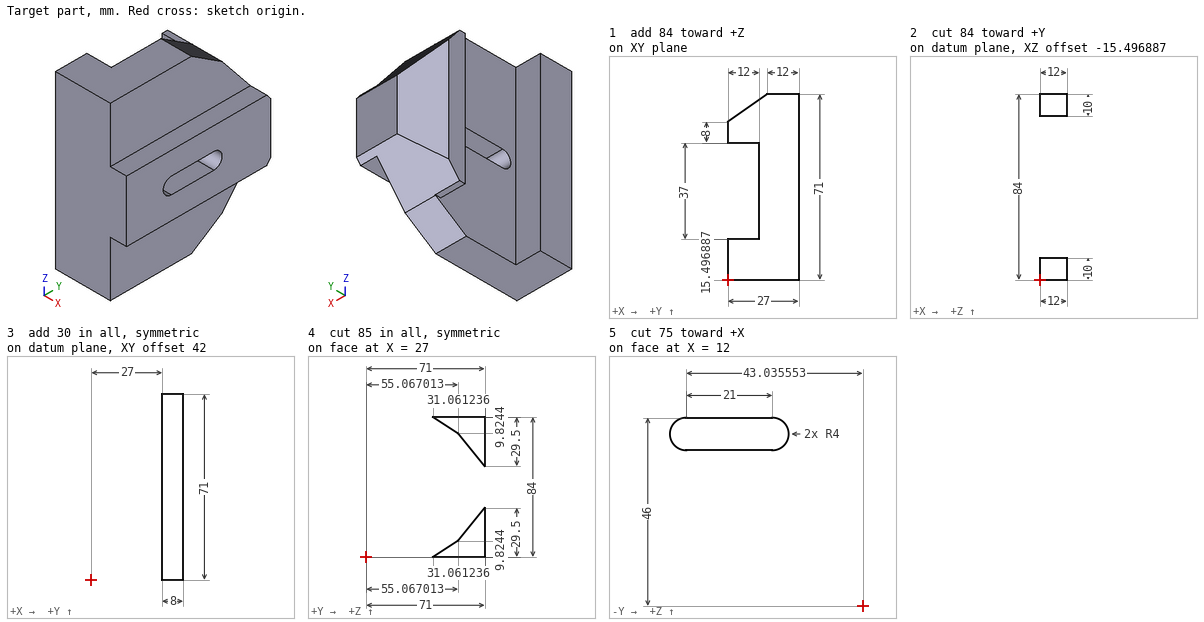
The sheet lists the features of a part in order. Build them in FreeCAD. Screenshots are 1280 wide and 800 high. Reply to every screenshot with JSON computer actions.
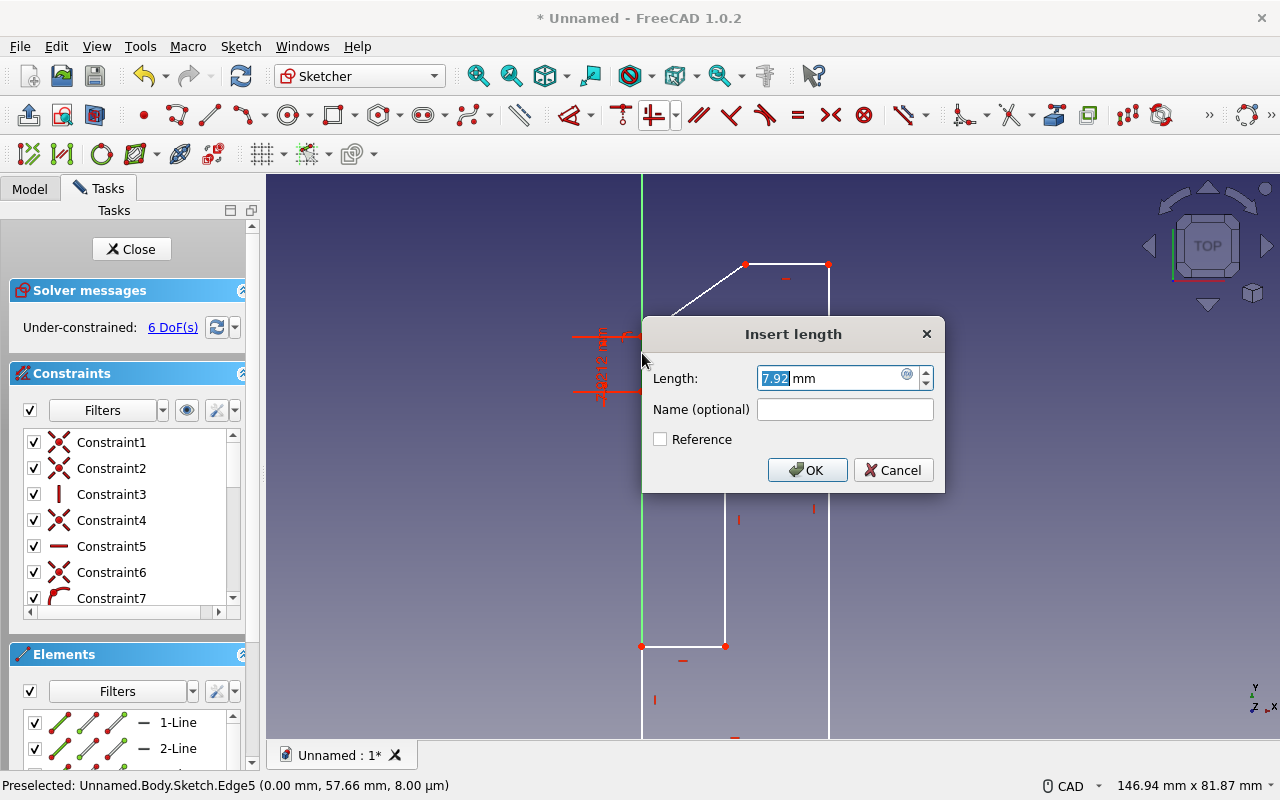
{"action": "type", "text": "8"}
{"action": "key", "text": "Return"}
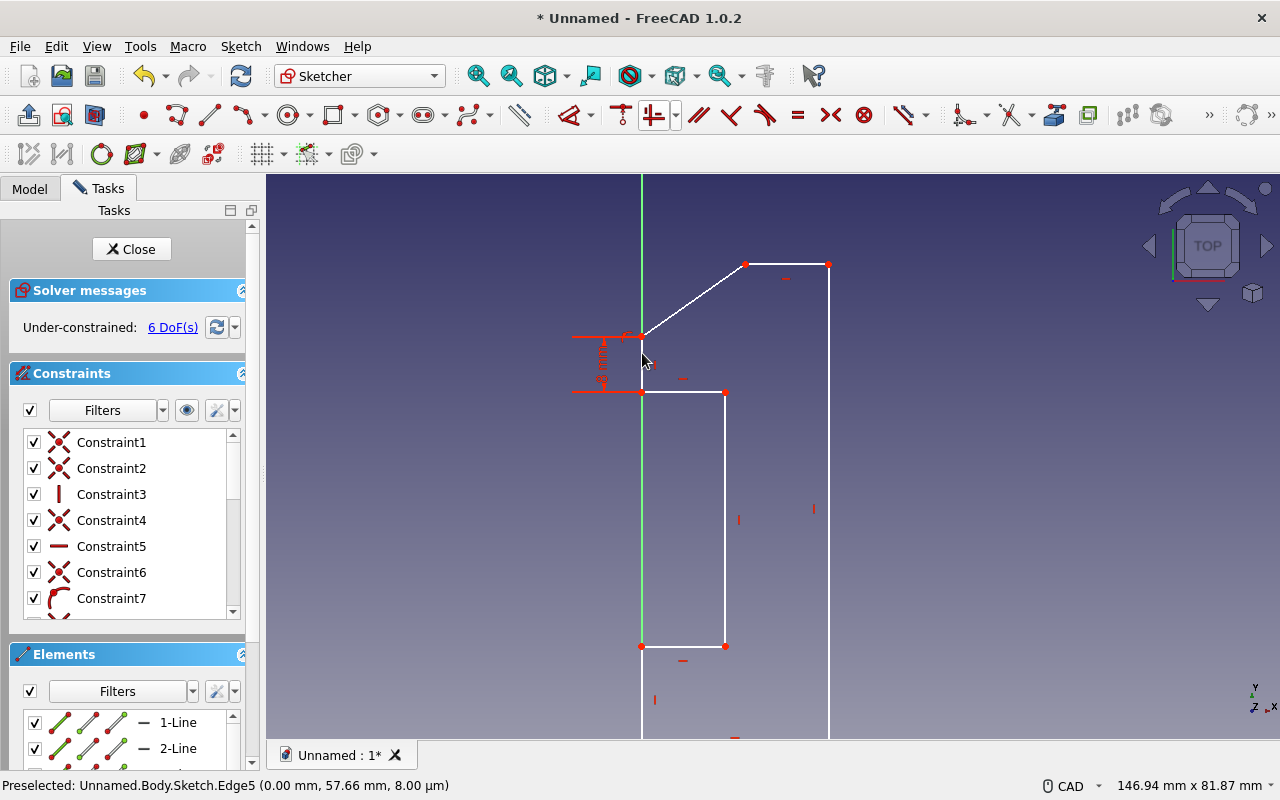
{"action": "scroll", "coordinate": [642, 354], "scroll_direction": "down", "scroll_amount": 2}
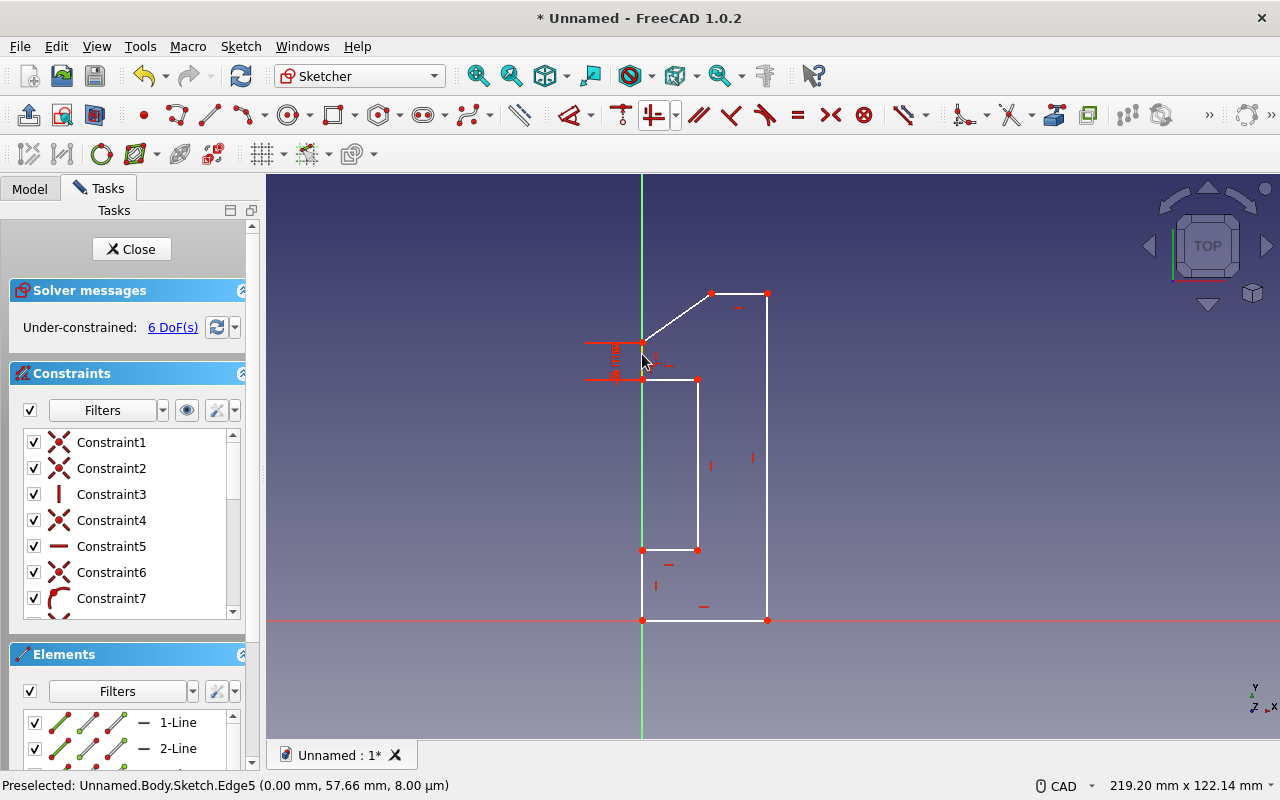
{"action": "left_click", "coordinate": [680, 621]}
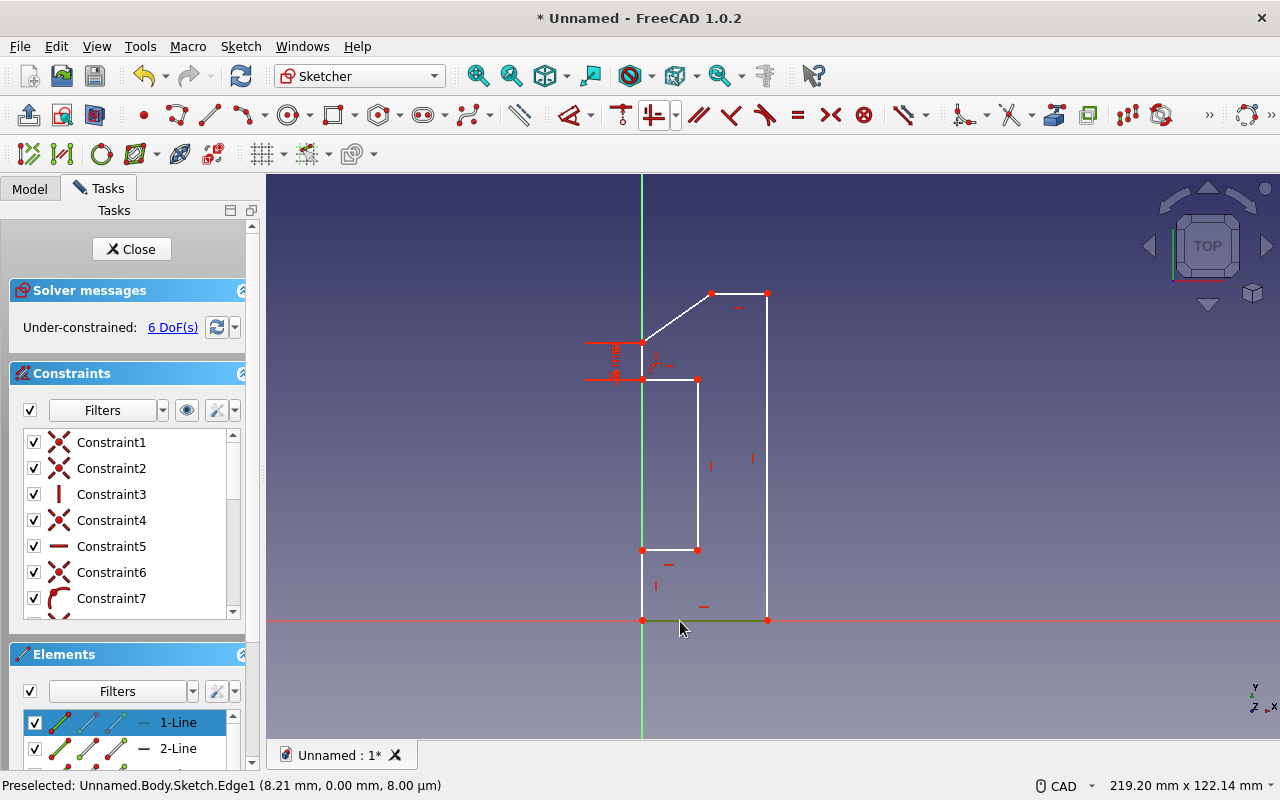
{"action": "key", "text": "l"}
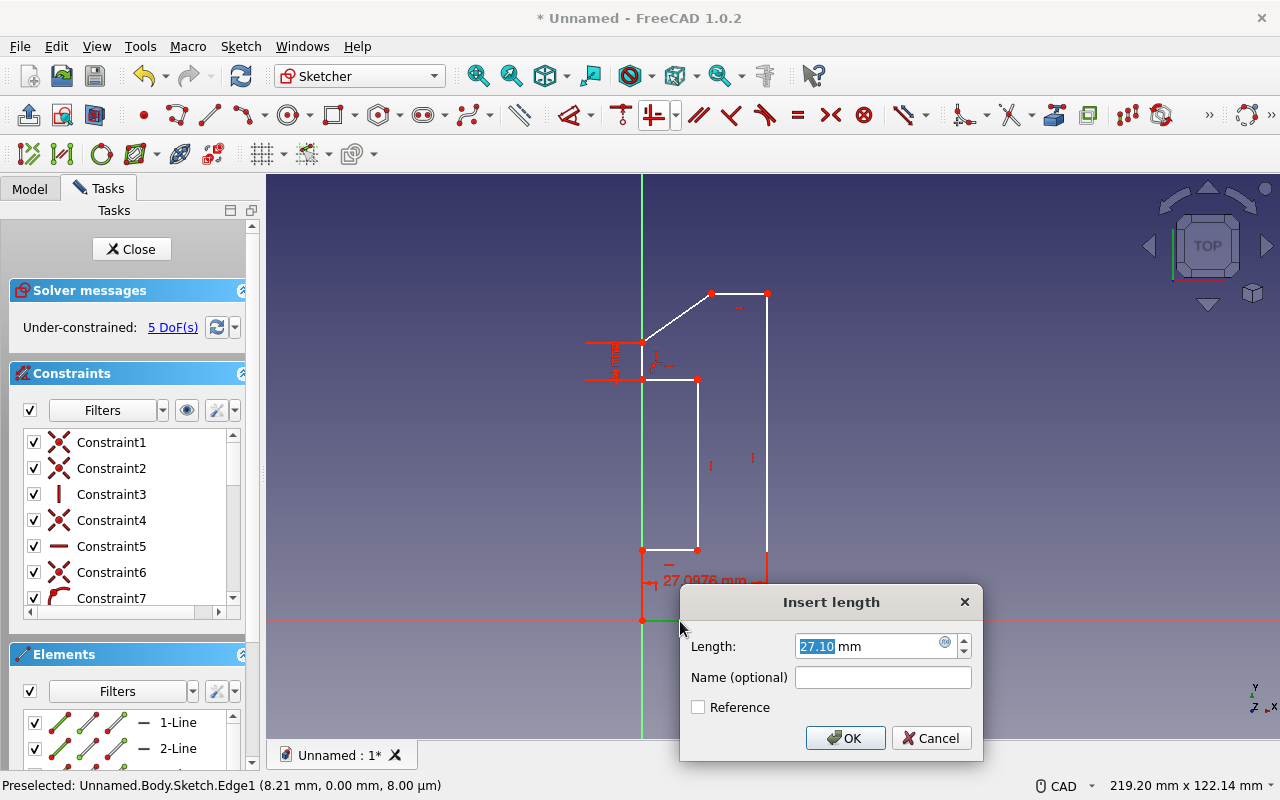
{"action": "type", "text": "27"}
{"action": "key", "text": "Return"}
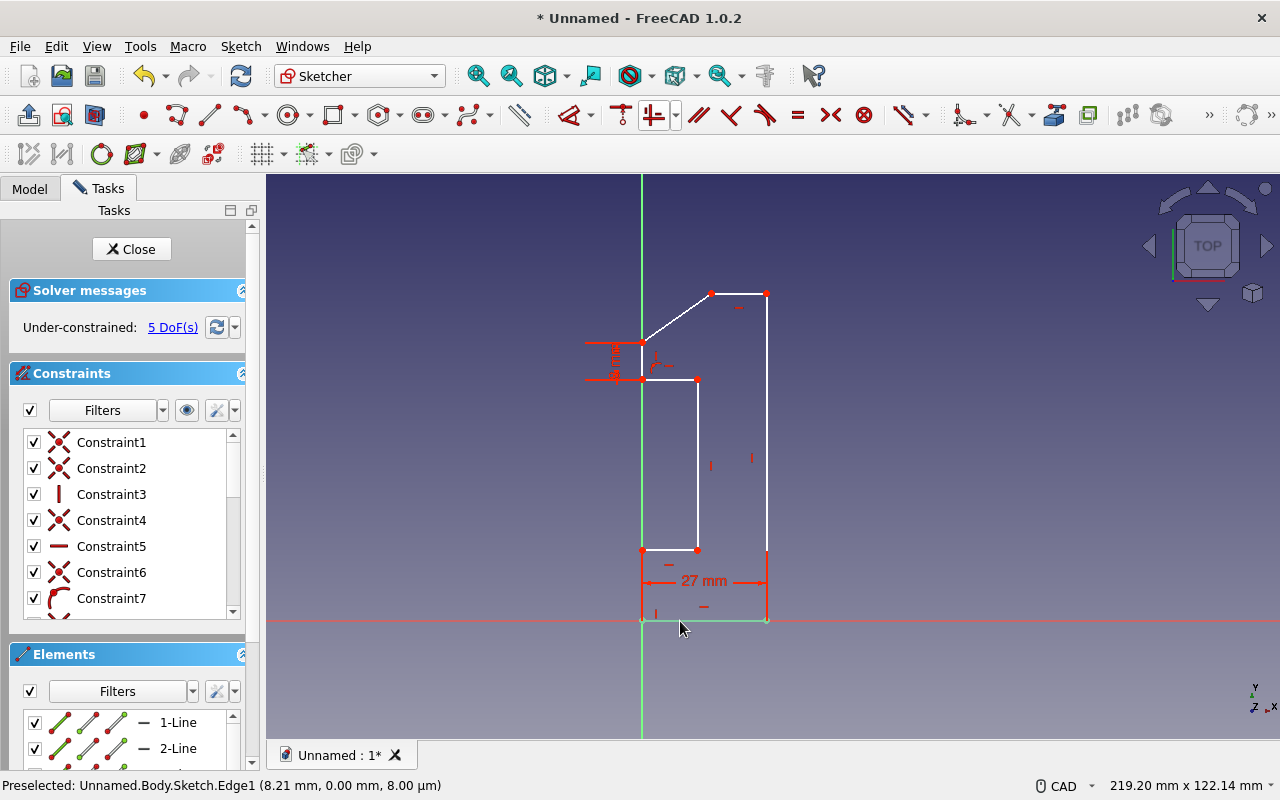
{"action": "left_click", "coordinate": [767, 523]}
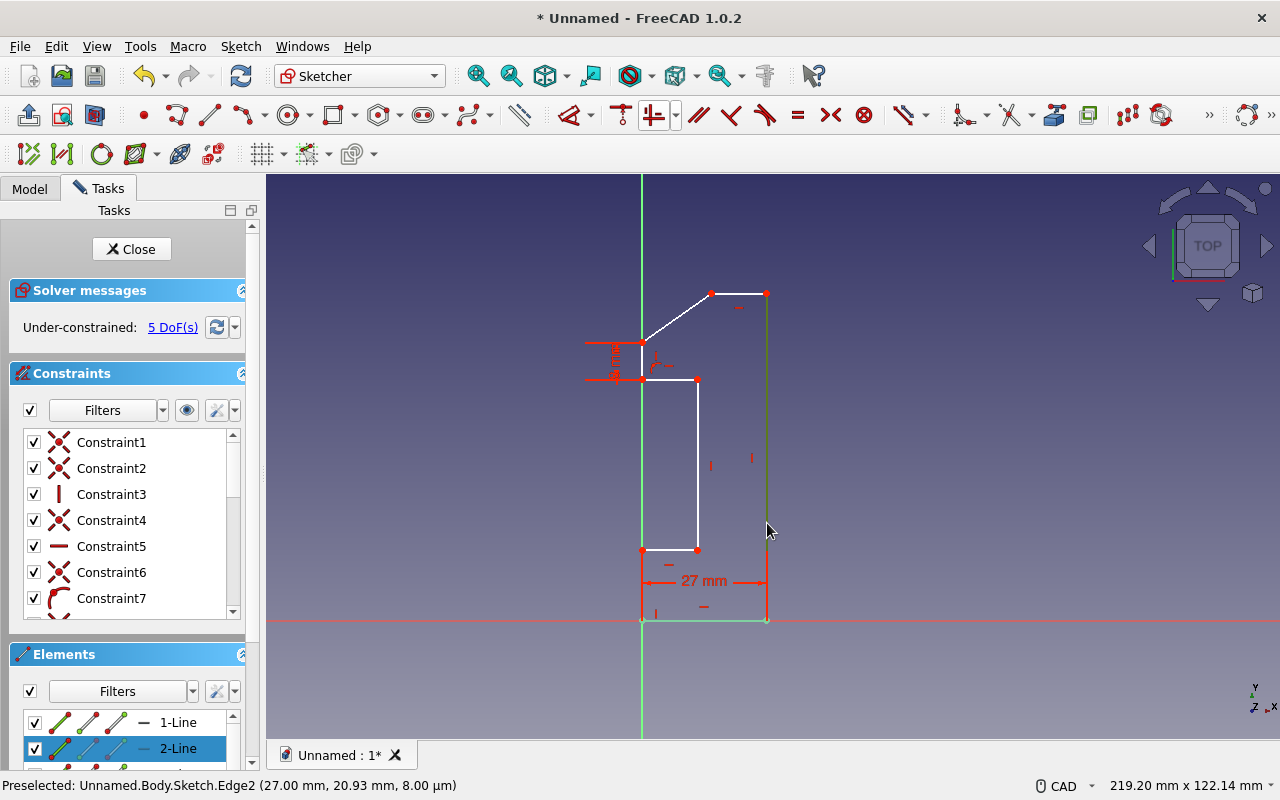
{"action": "left_click", "coordinate": [590, 116]}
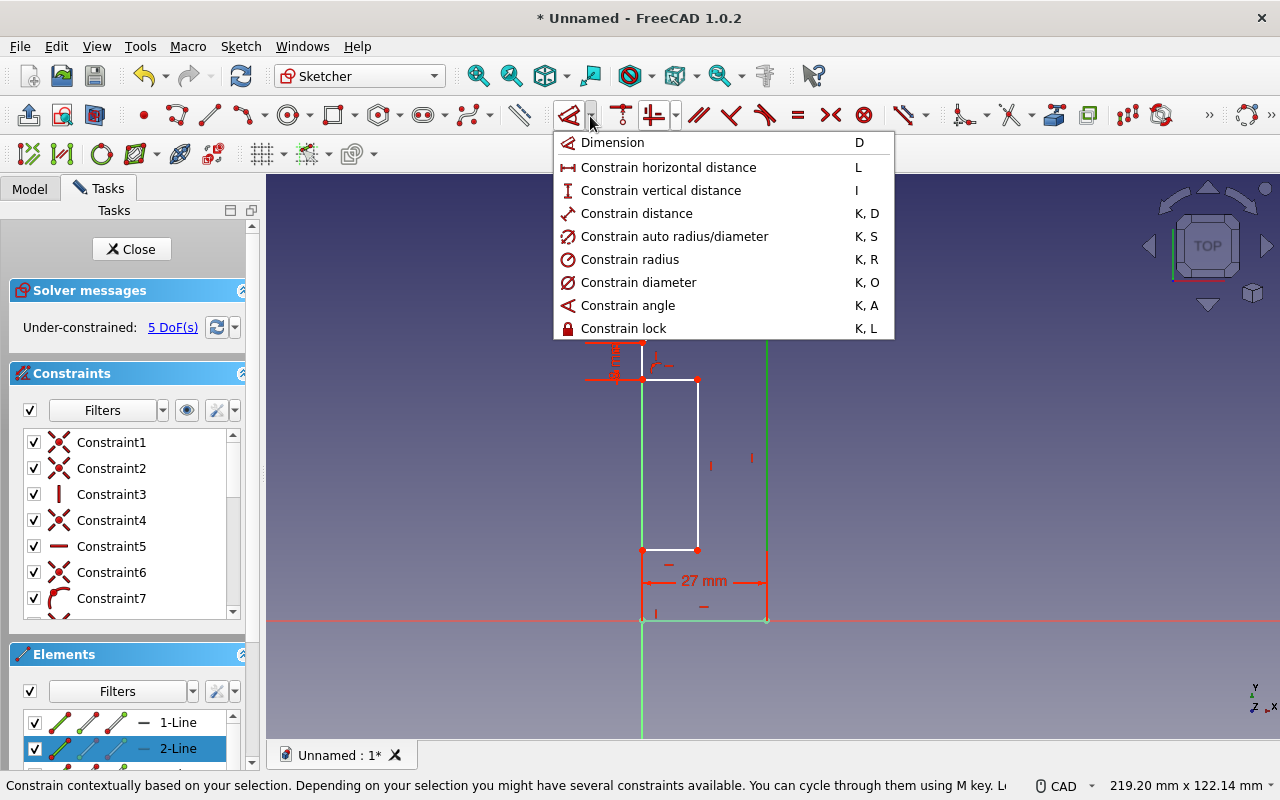
{"action": "left_click", "coordinate": [724, 190]}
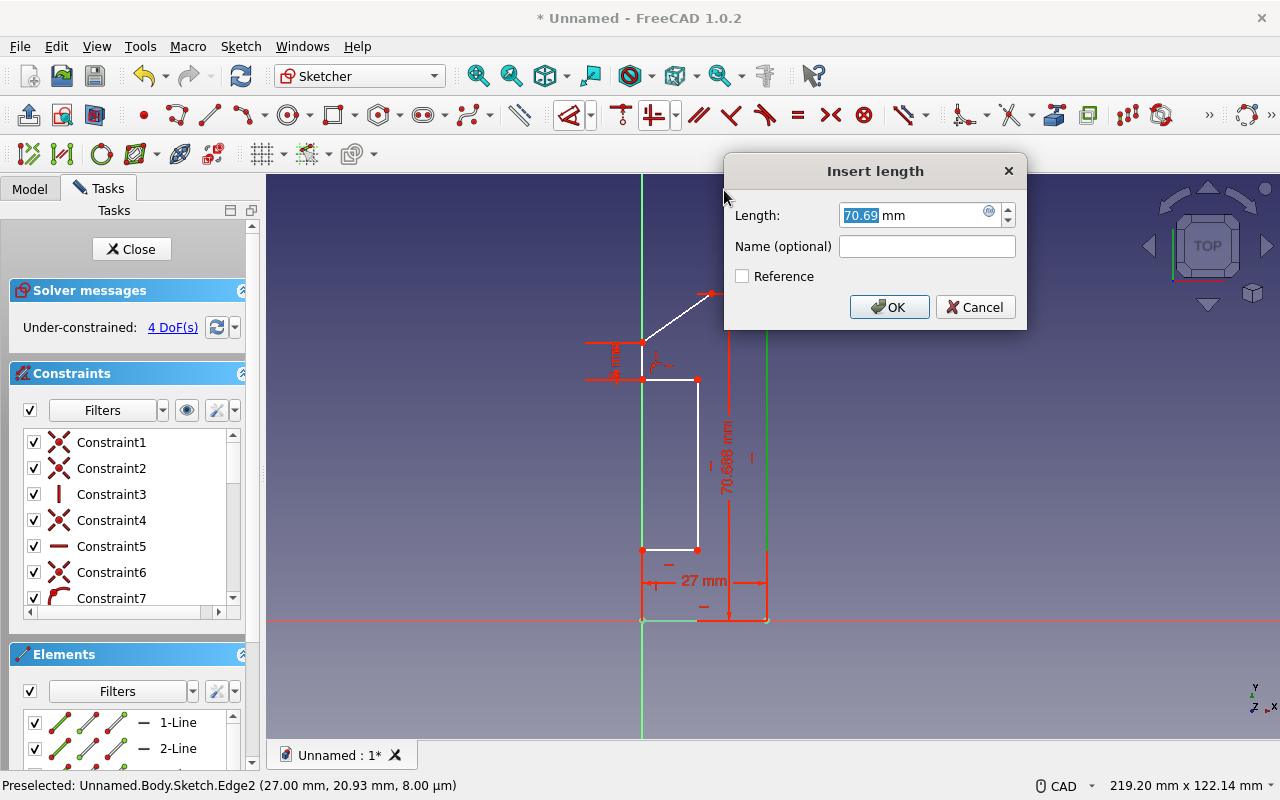
{"action": "type", "text": "71"}
{"action": "key", "text": "Return"}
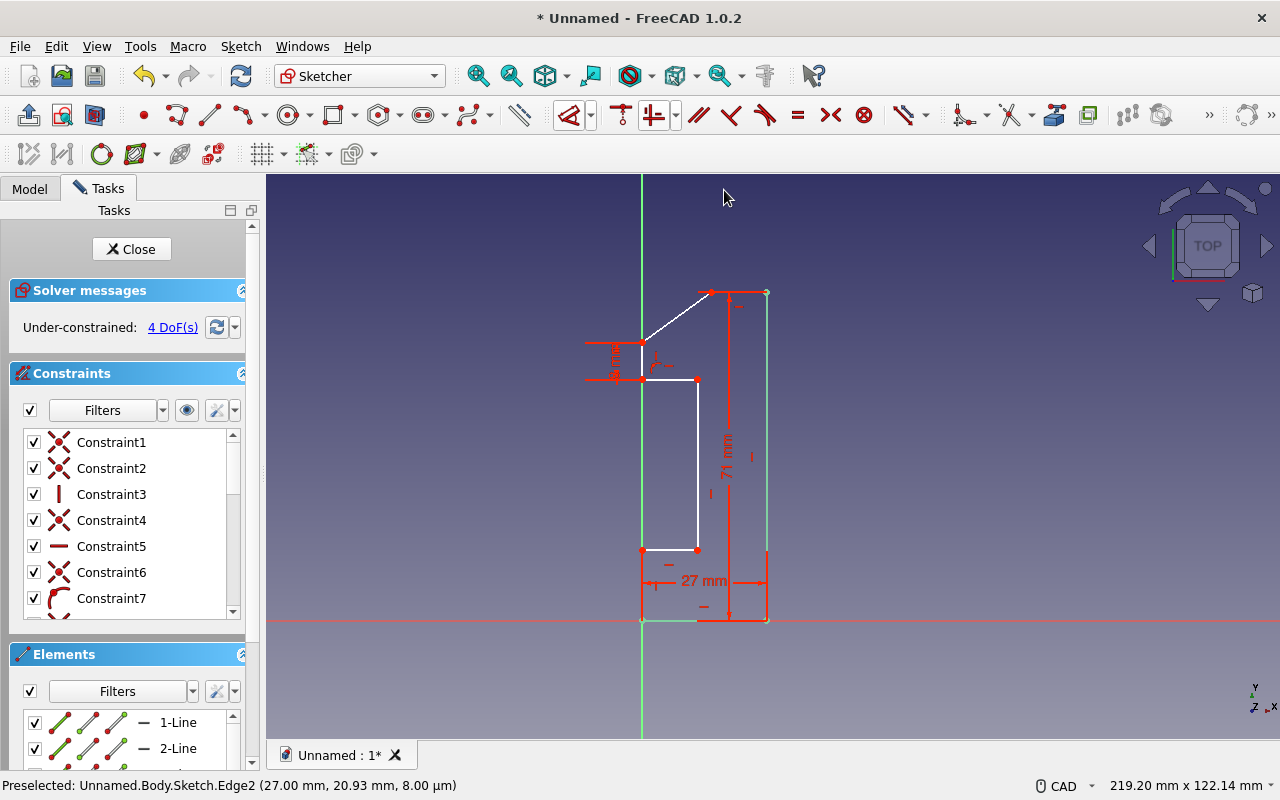
{"action": "left_click", "coordinate": [750, 292]}